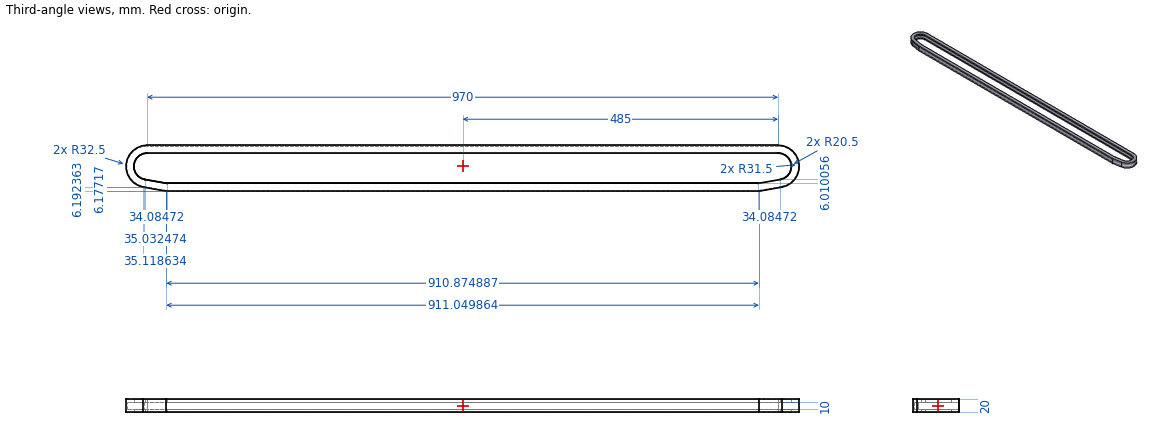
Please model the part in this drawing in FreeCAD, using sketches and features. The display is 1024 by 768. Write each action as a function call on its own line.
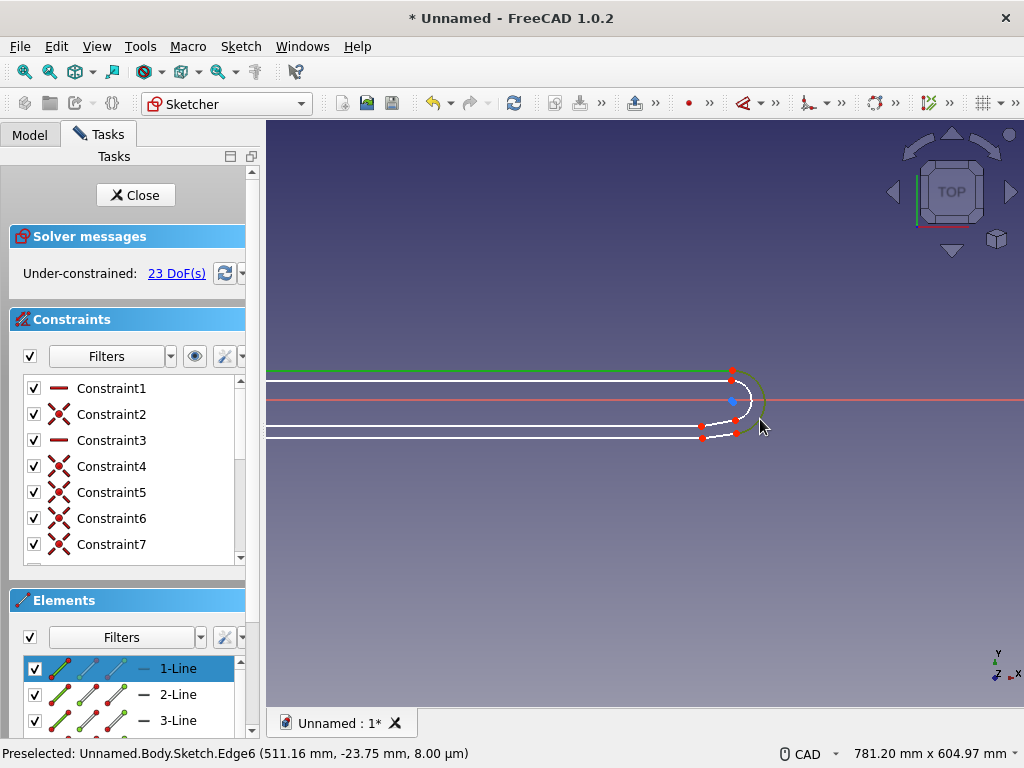
key(t)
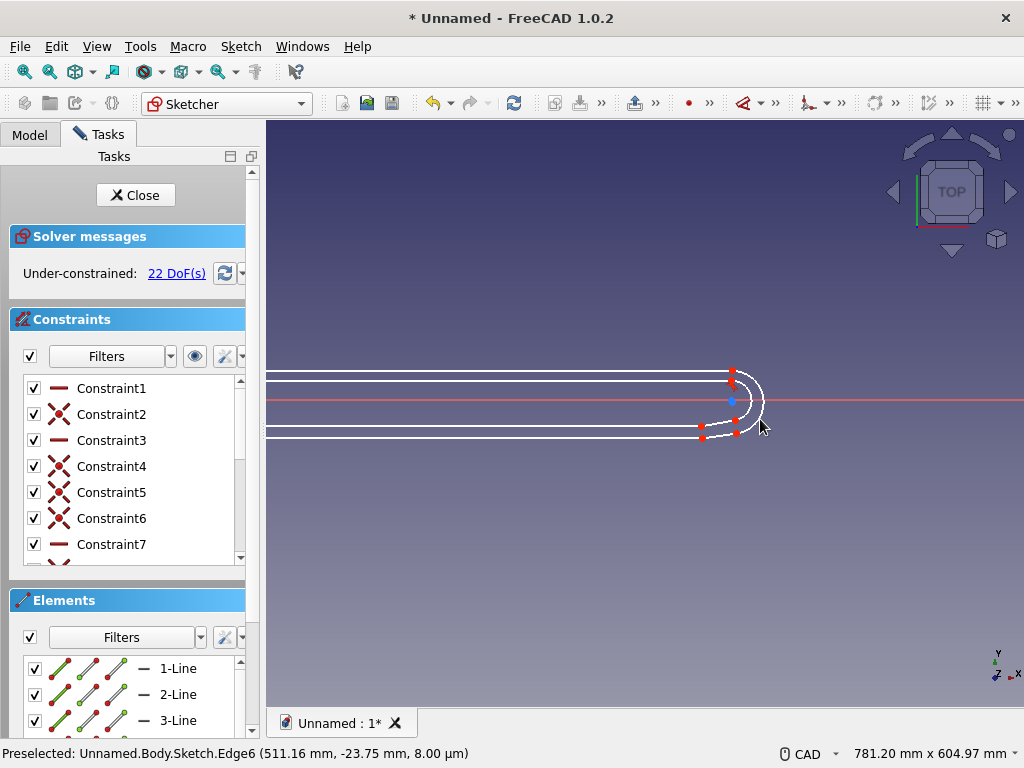
scroll(760, 420, down, 5)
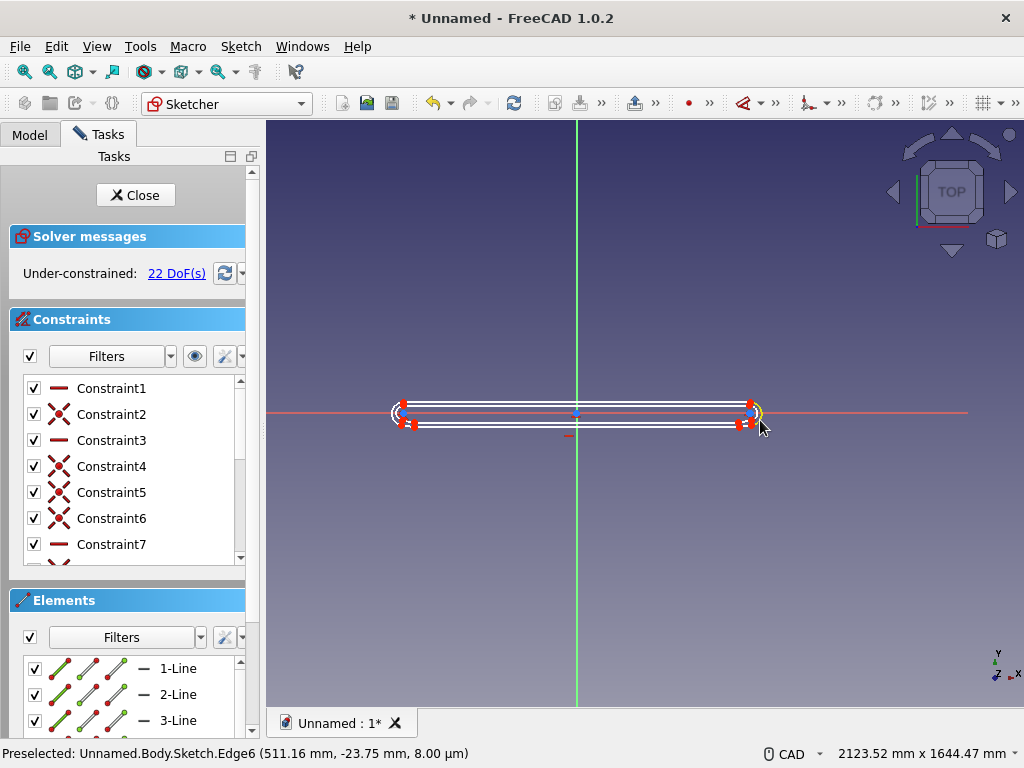
scroll(405, 426, up, 7)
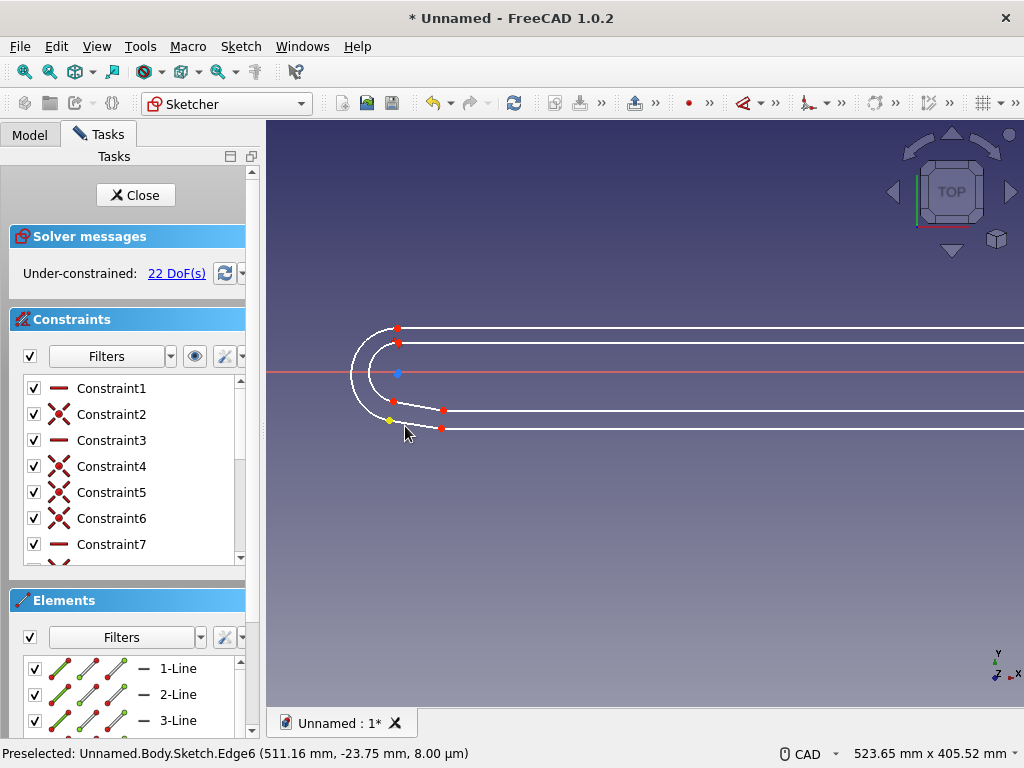
click(405, 423)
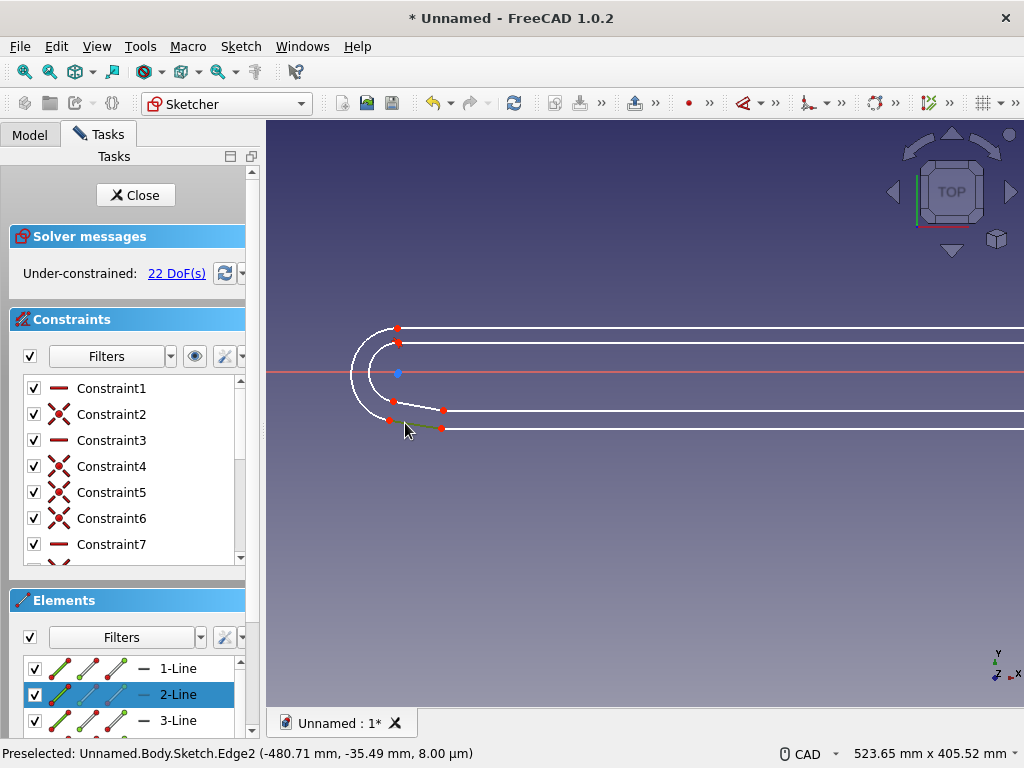
click(362, 345)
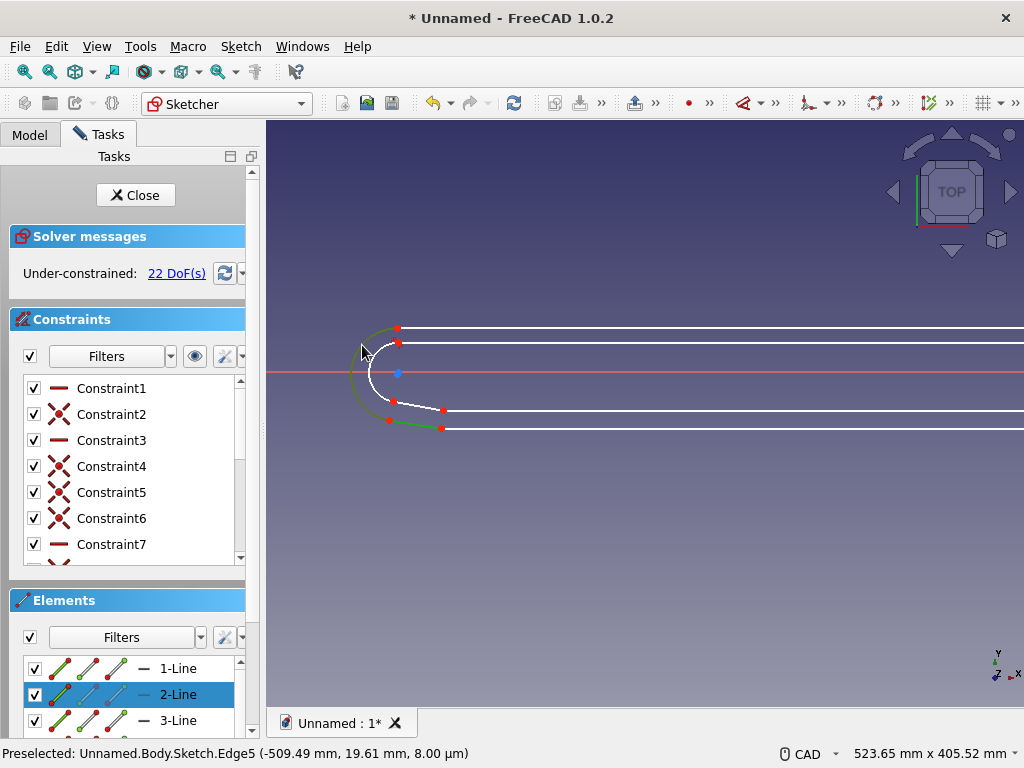
key(t)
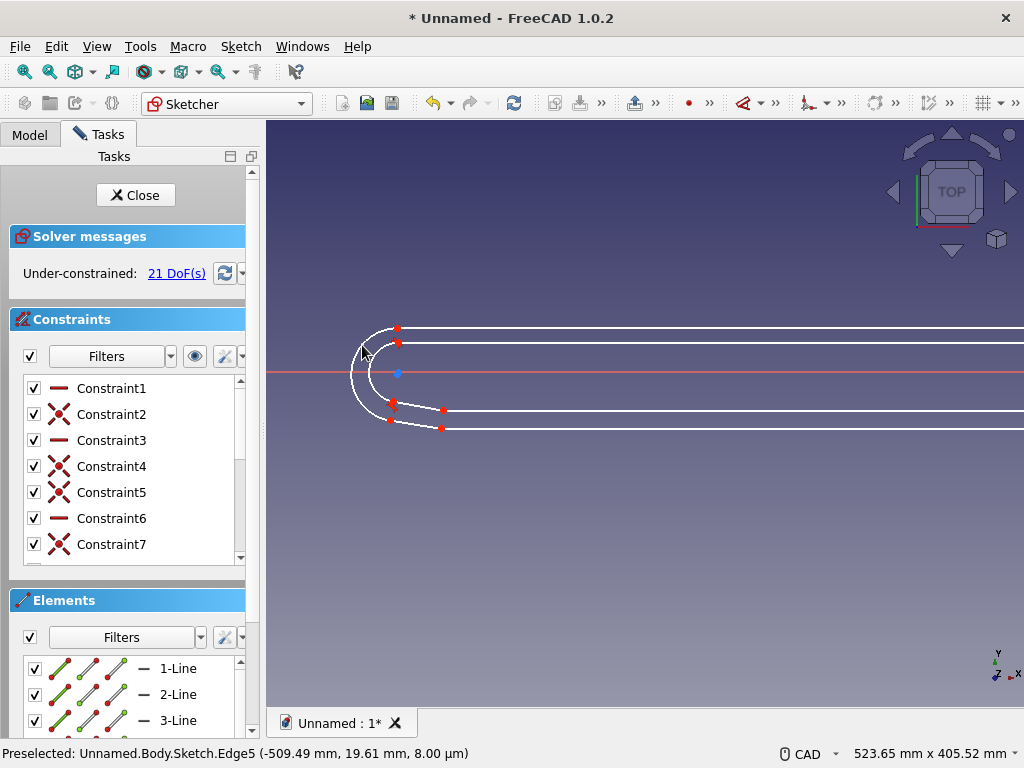
scroll(405, 426, down, 7)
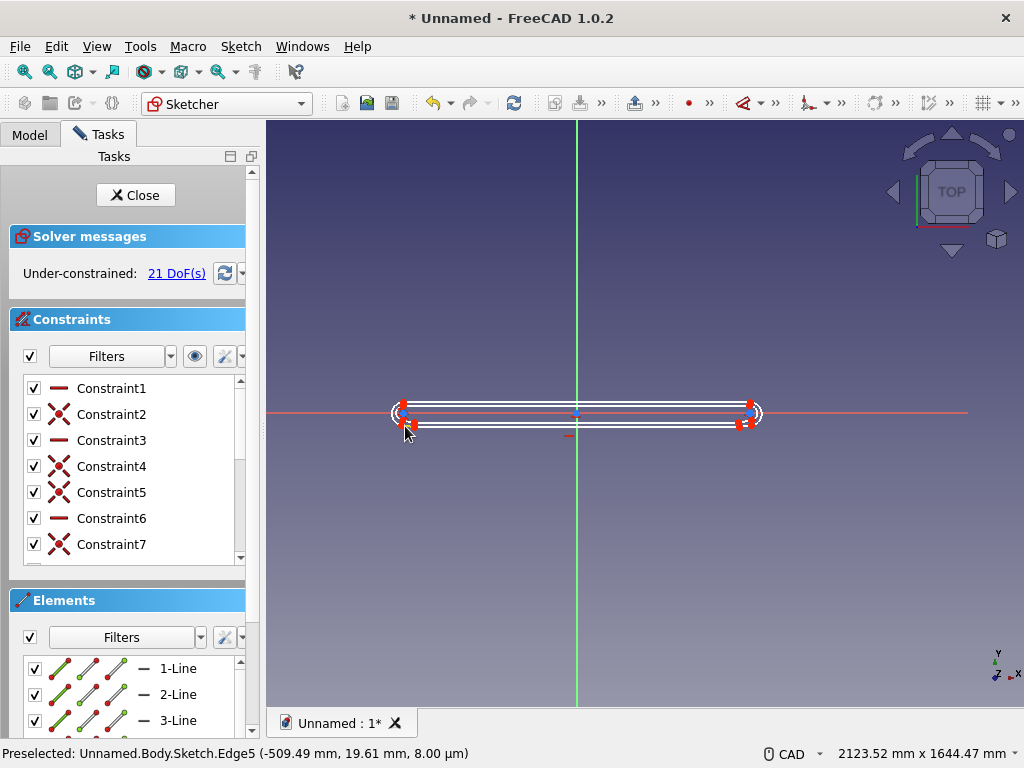
scroll(743, 427, up, 7)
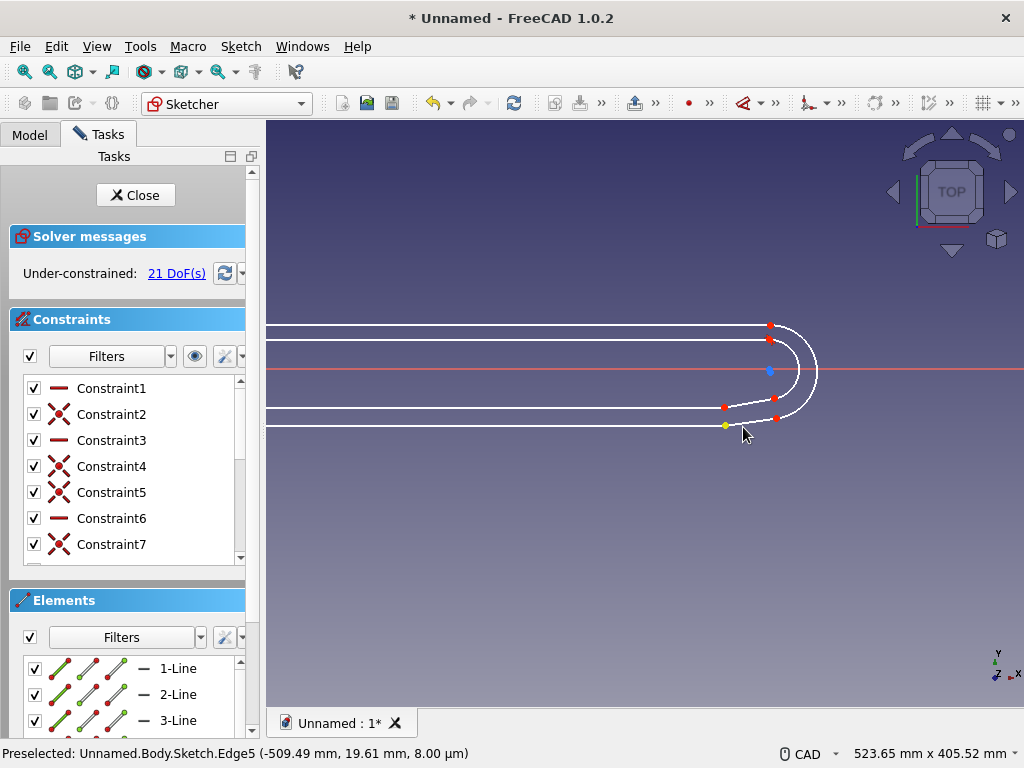
click(741, 424)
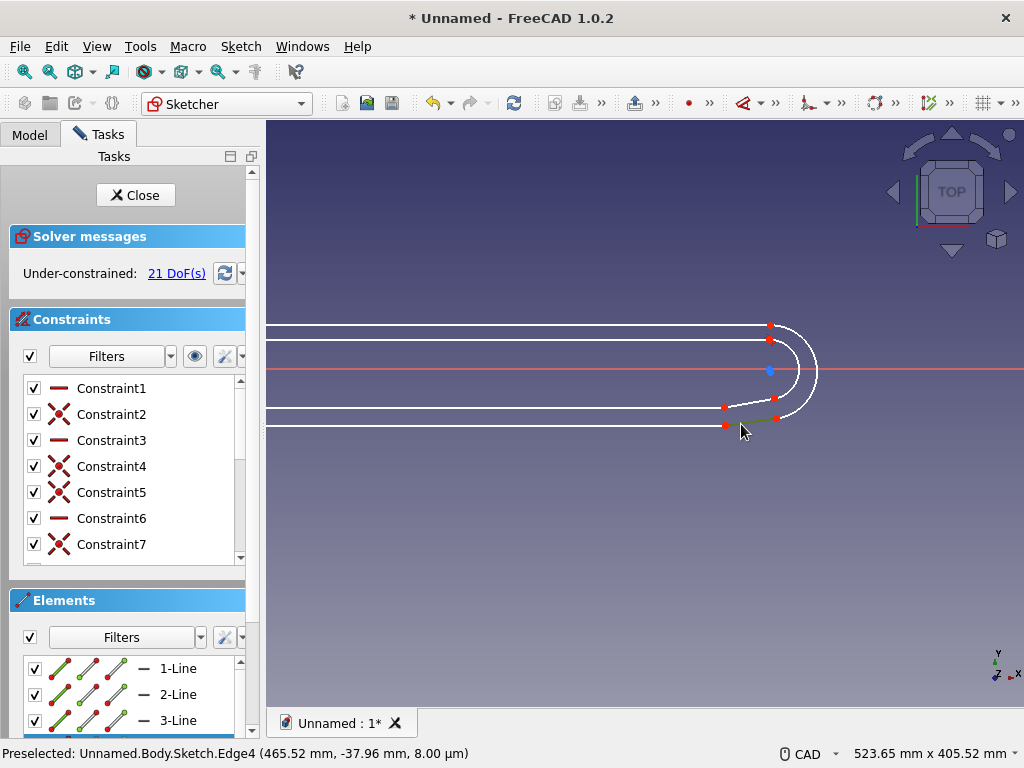
click(811, 396)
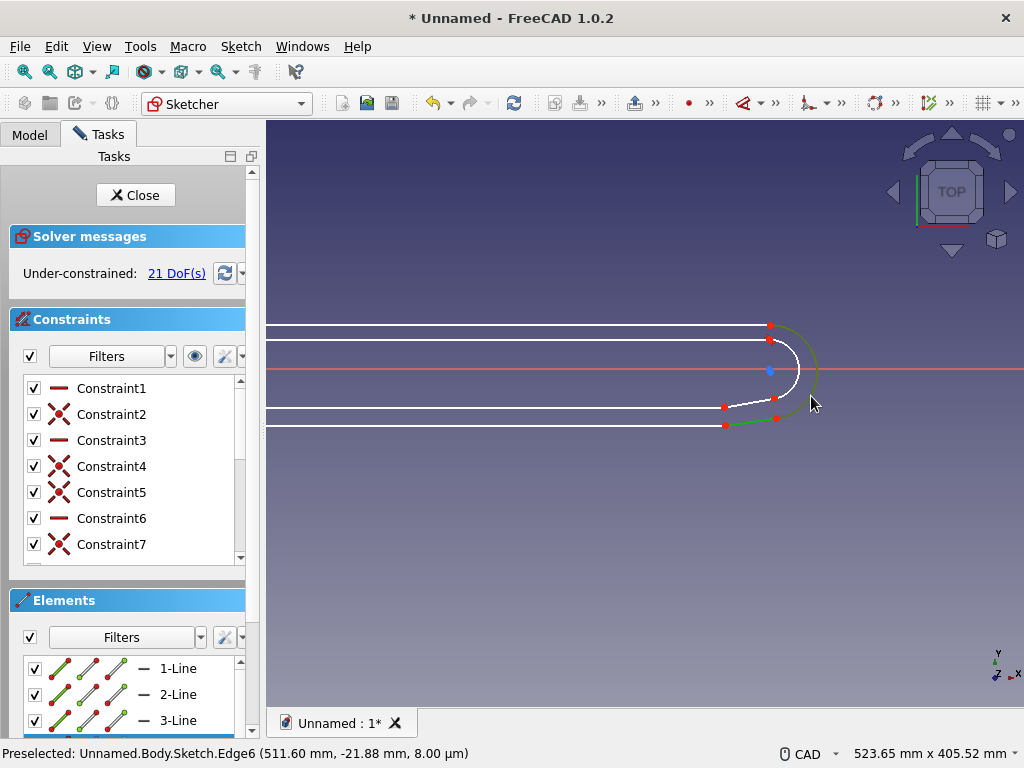
key(t)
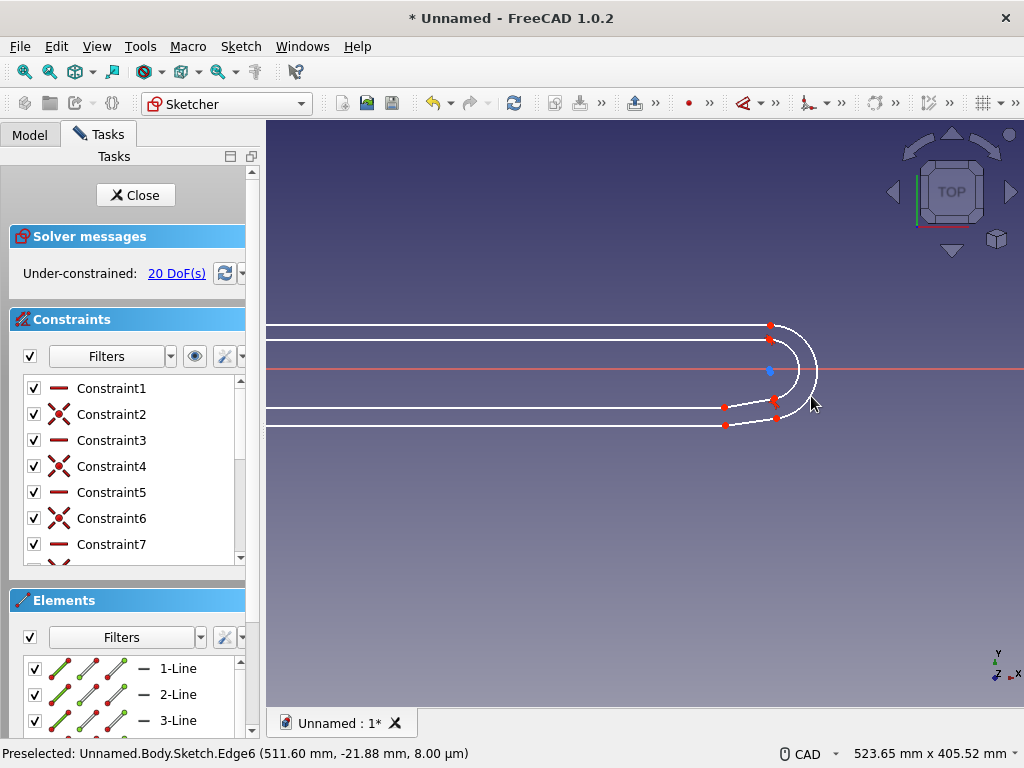
click(348, 340)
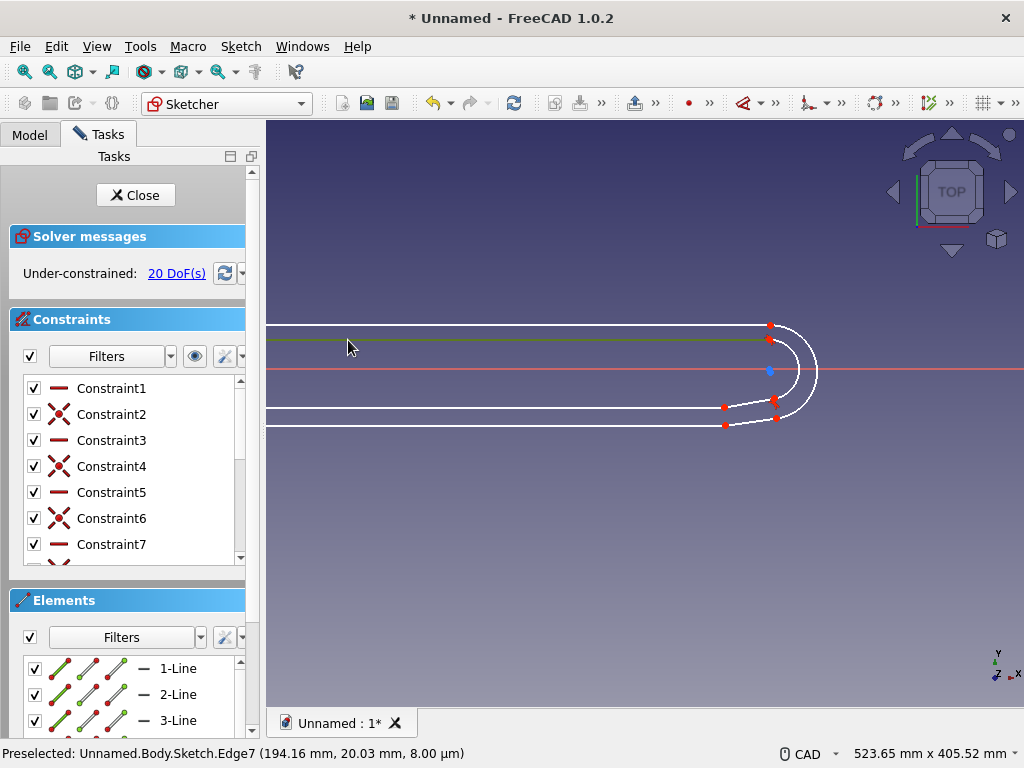
click(795, 384)